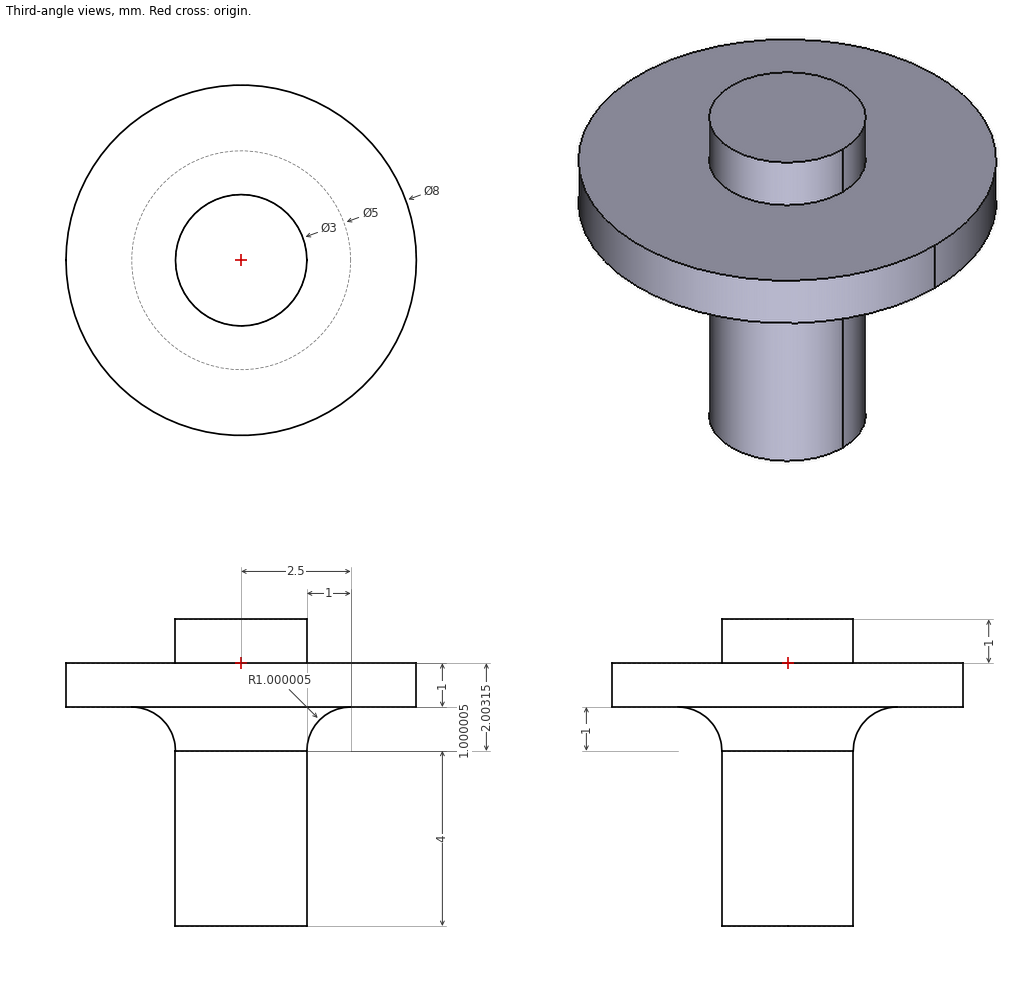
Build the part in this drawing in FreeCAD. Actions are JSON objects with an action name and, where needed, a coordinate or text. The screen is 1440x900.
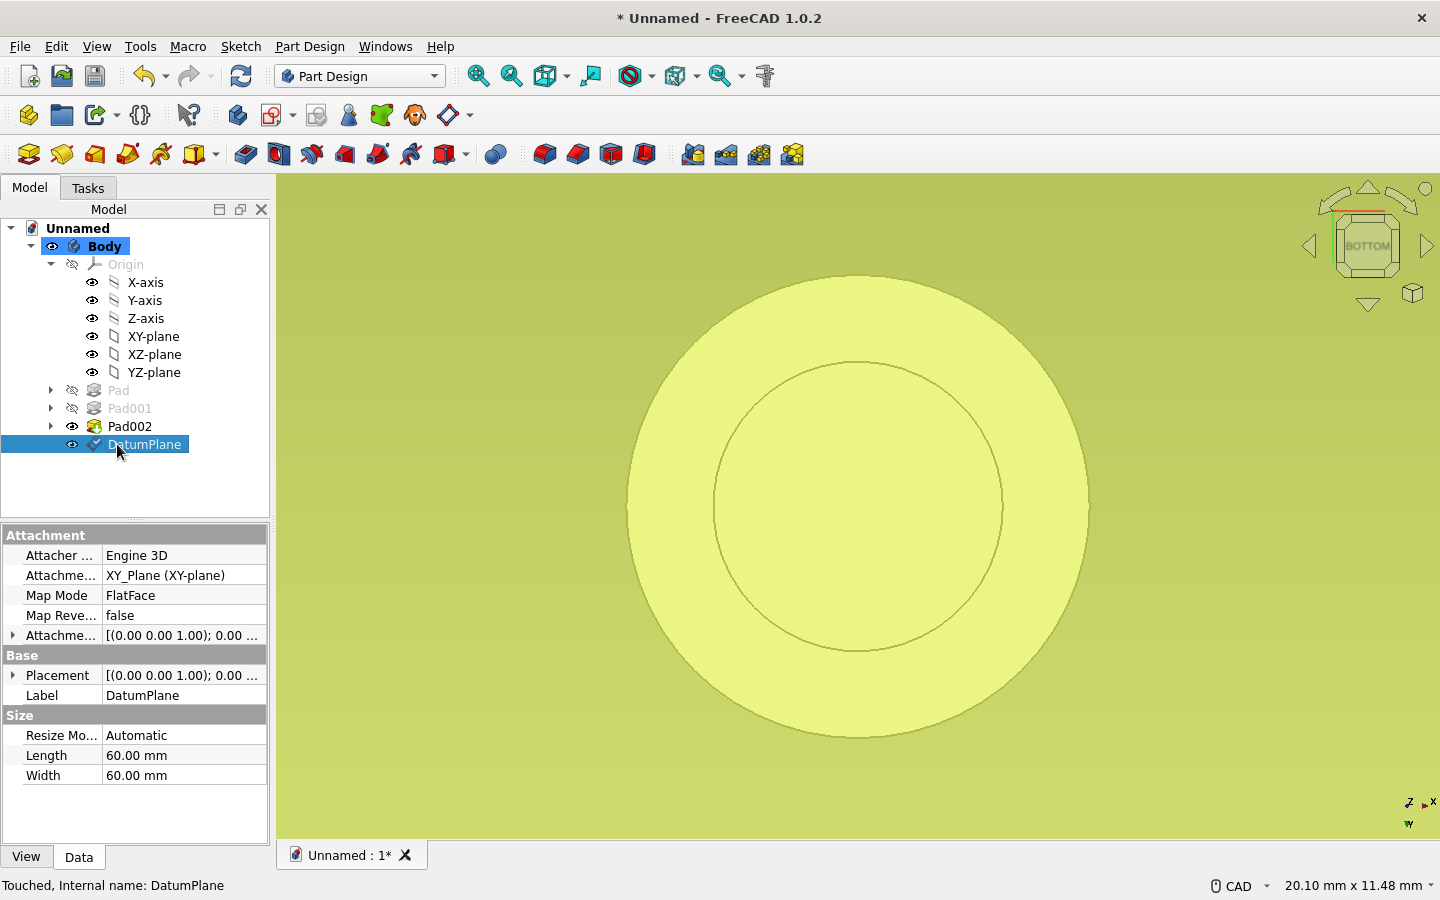
{"action": "left_click", "coordinate": [270, 116]}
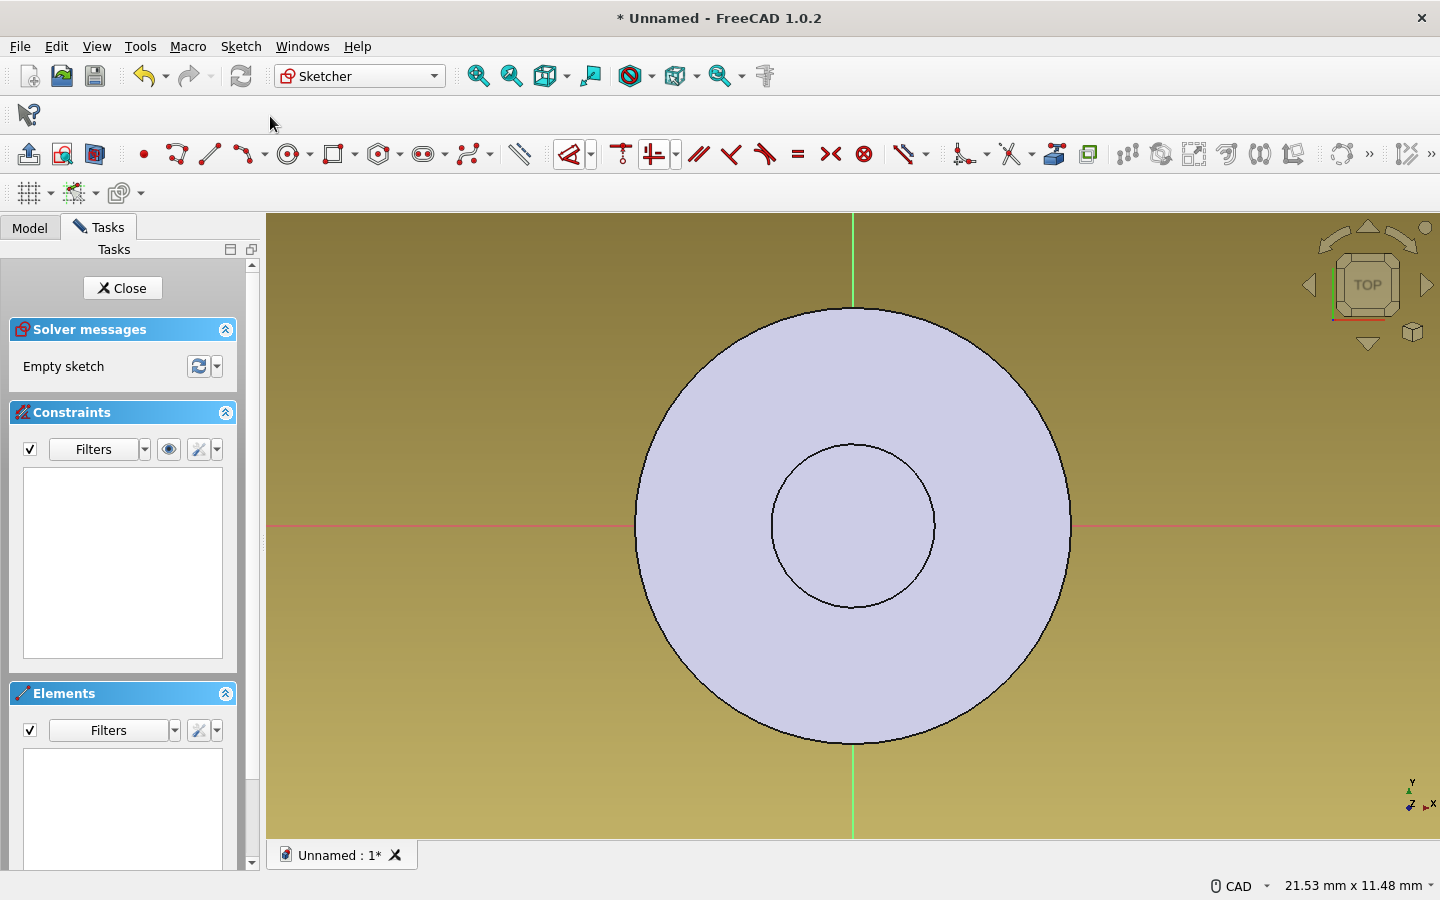
{"action": "left_click", "coordinate": [95, 154]}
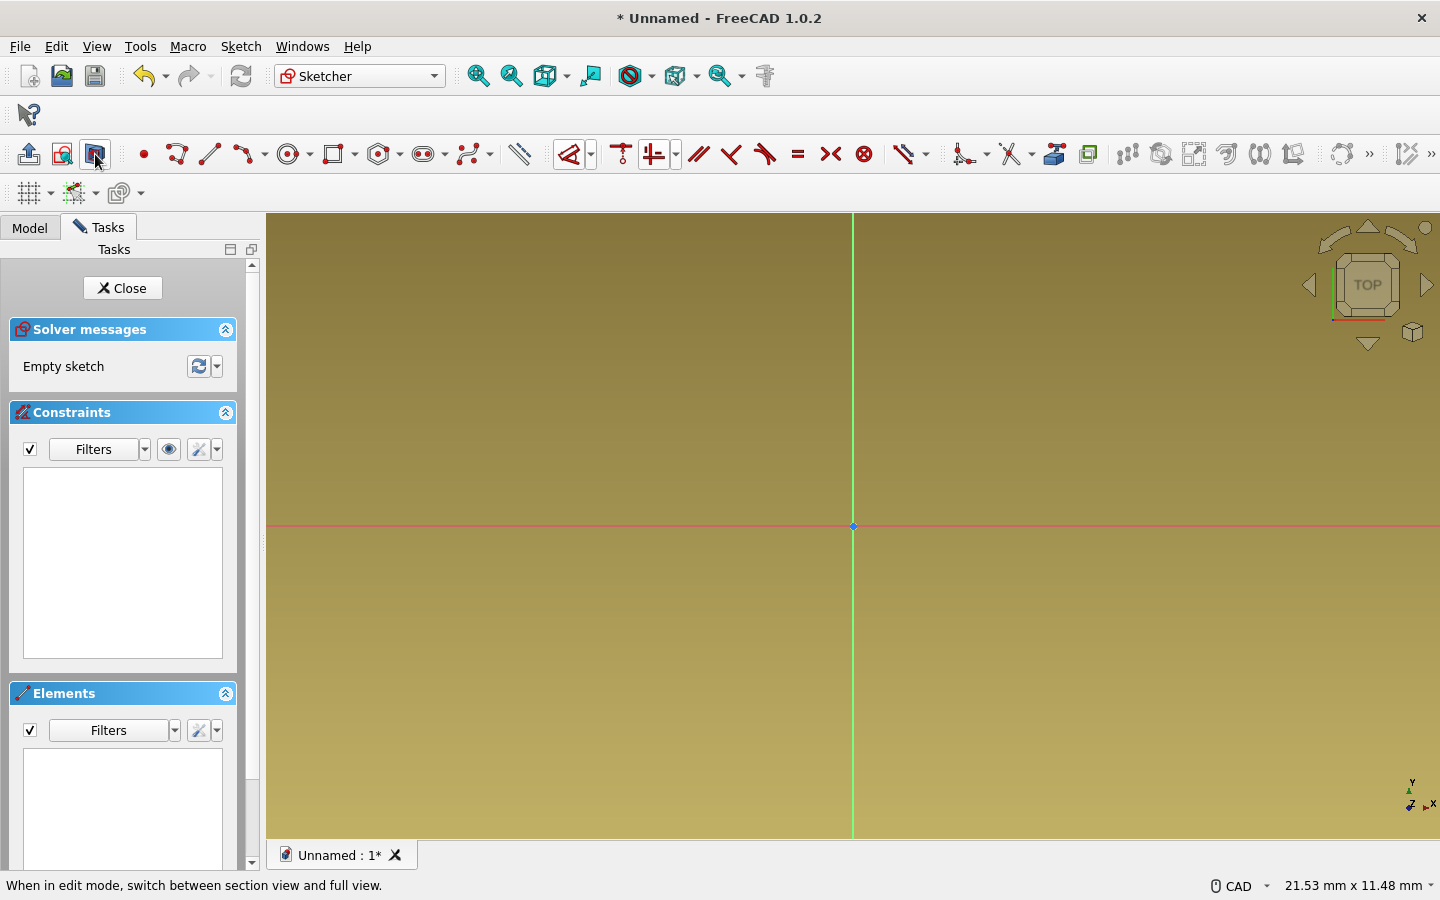
{"action": "scroll", "coordinate": [909, 526], "scroll_direction": "up", "scroll_amount": 4}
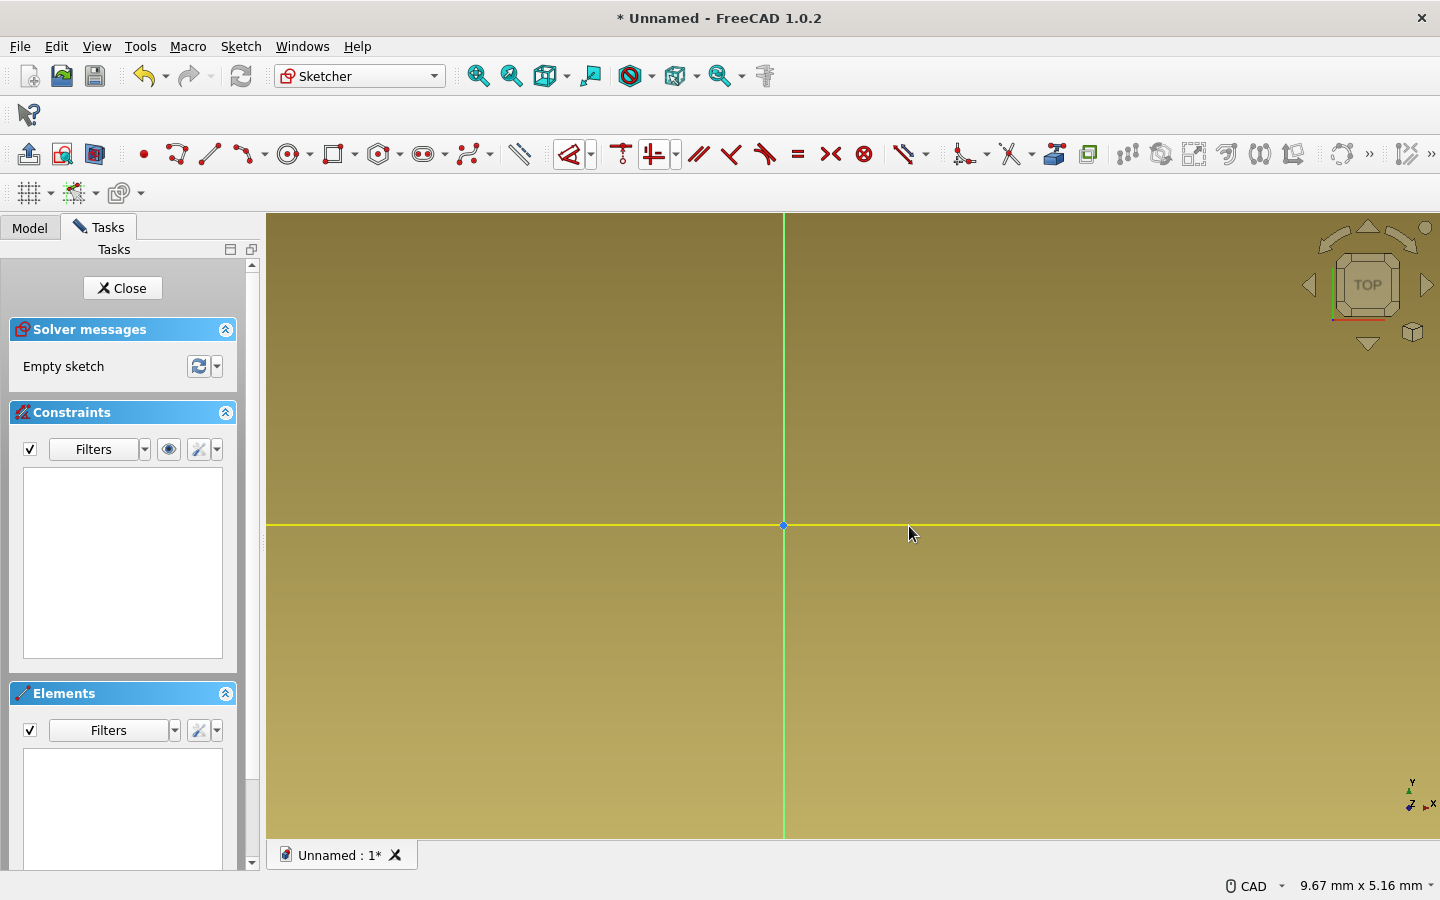
{"action": "left_click", "coordinate": [288, 154]}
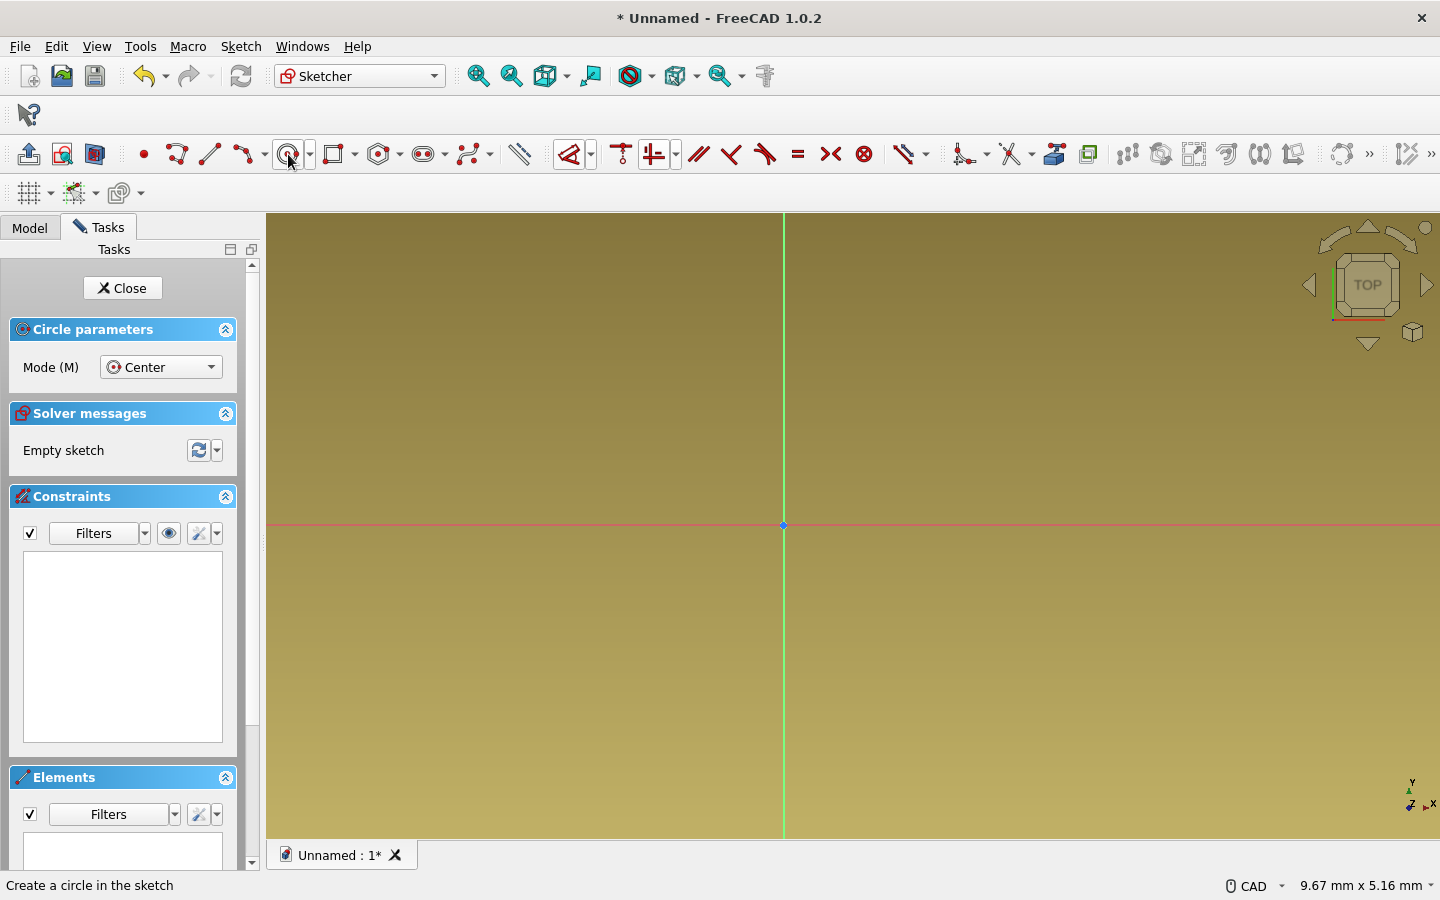
{"action": "left_click", "coordinate": [784, 525]}
{"action": "left_click", "coordinate": [912, 397]}
{"action": "key", "text": "Escape"}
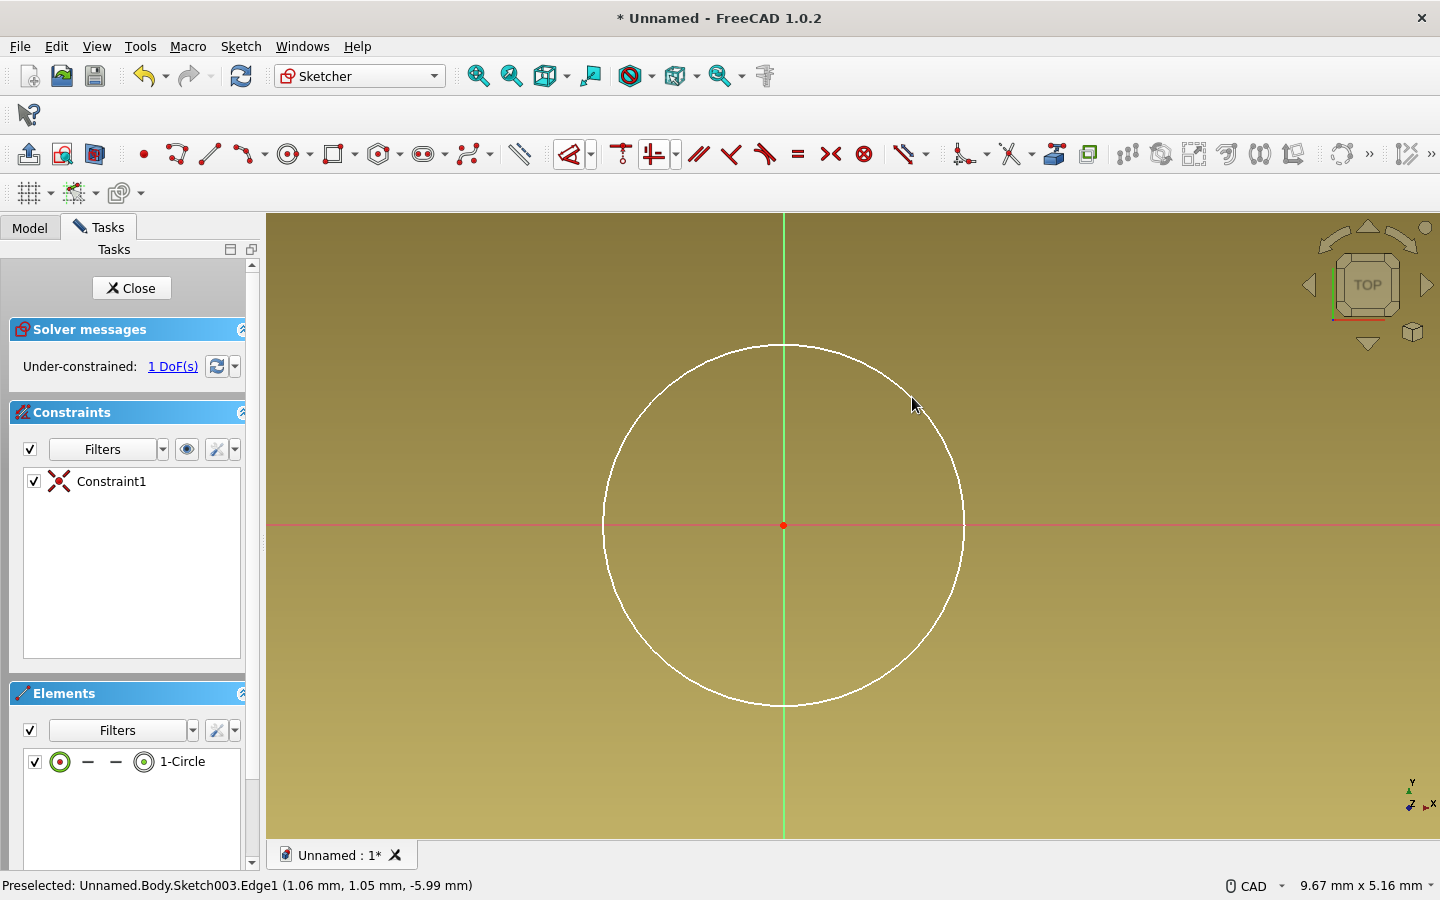
{"action": "left_click", "coordinate": [911, 397]}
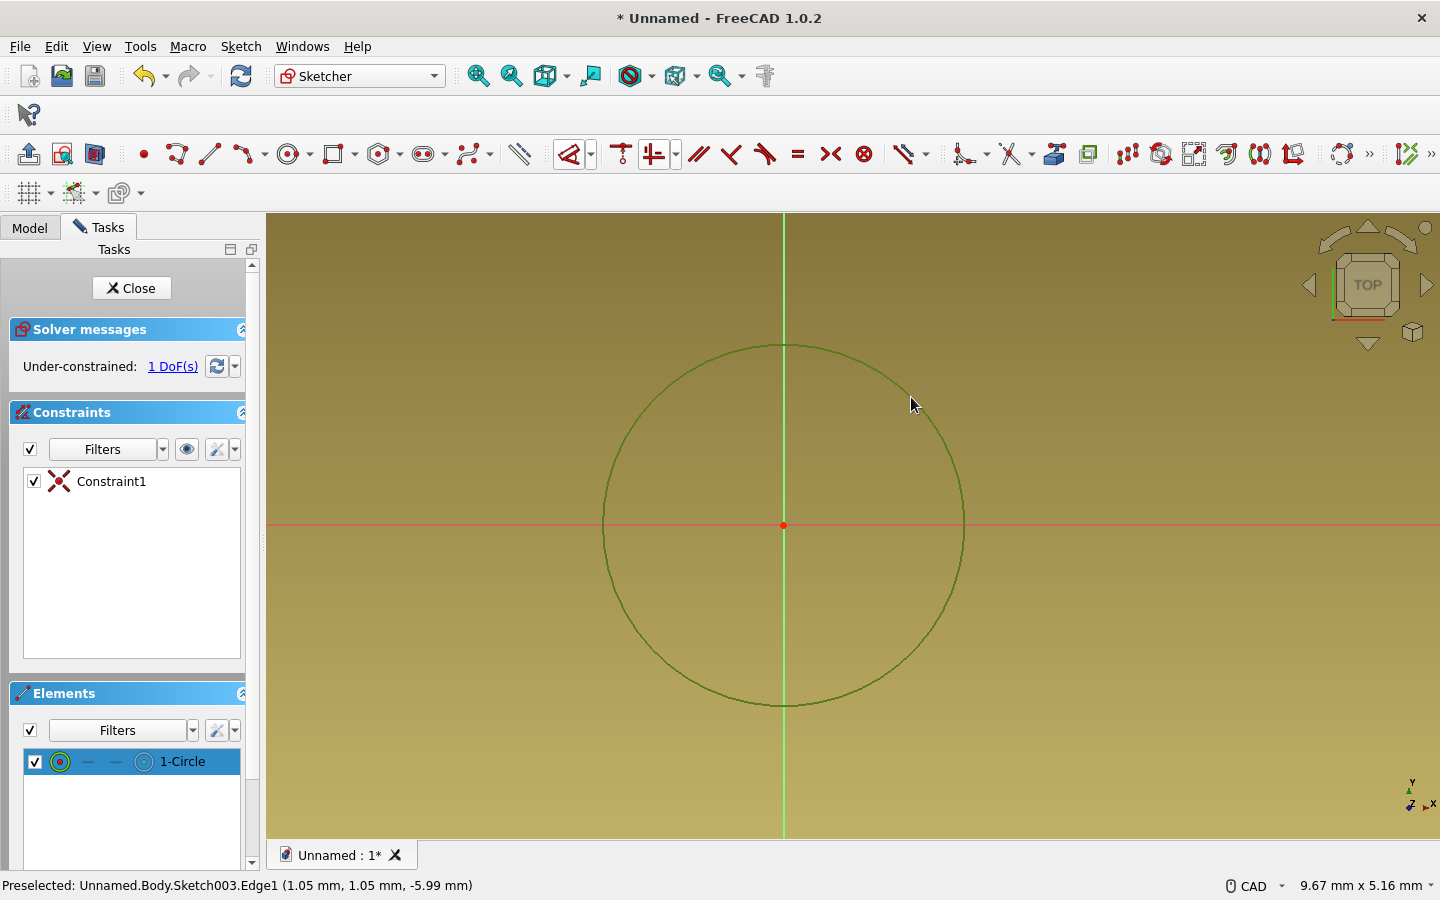
{"action": "left_click", "coordinate": [590, 154]}